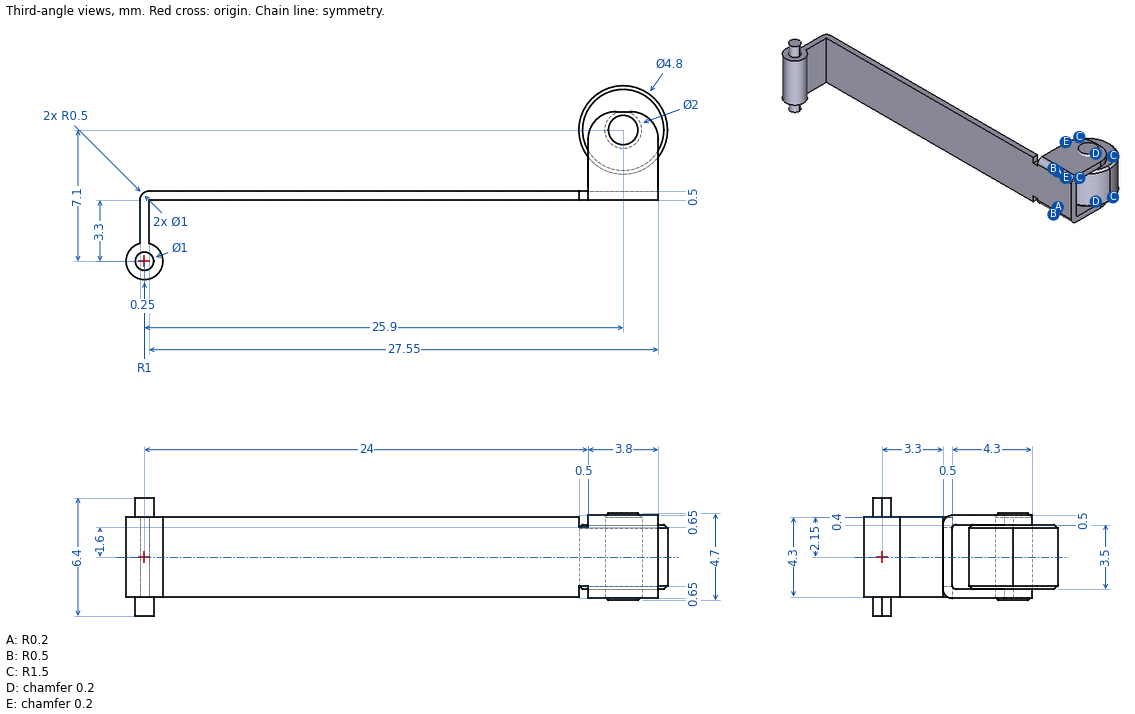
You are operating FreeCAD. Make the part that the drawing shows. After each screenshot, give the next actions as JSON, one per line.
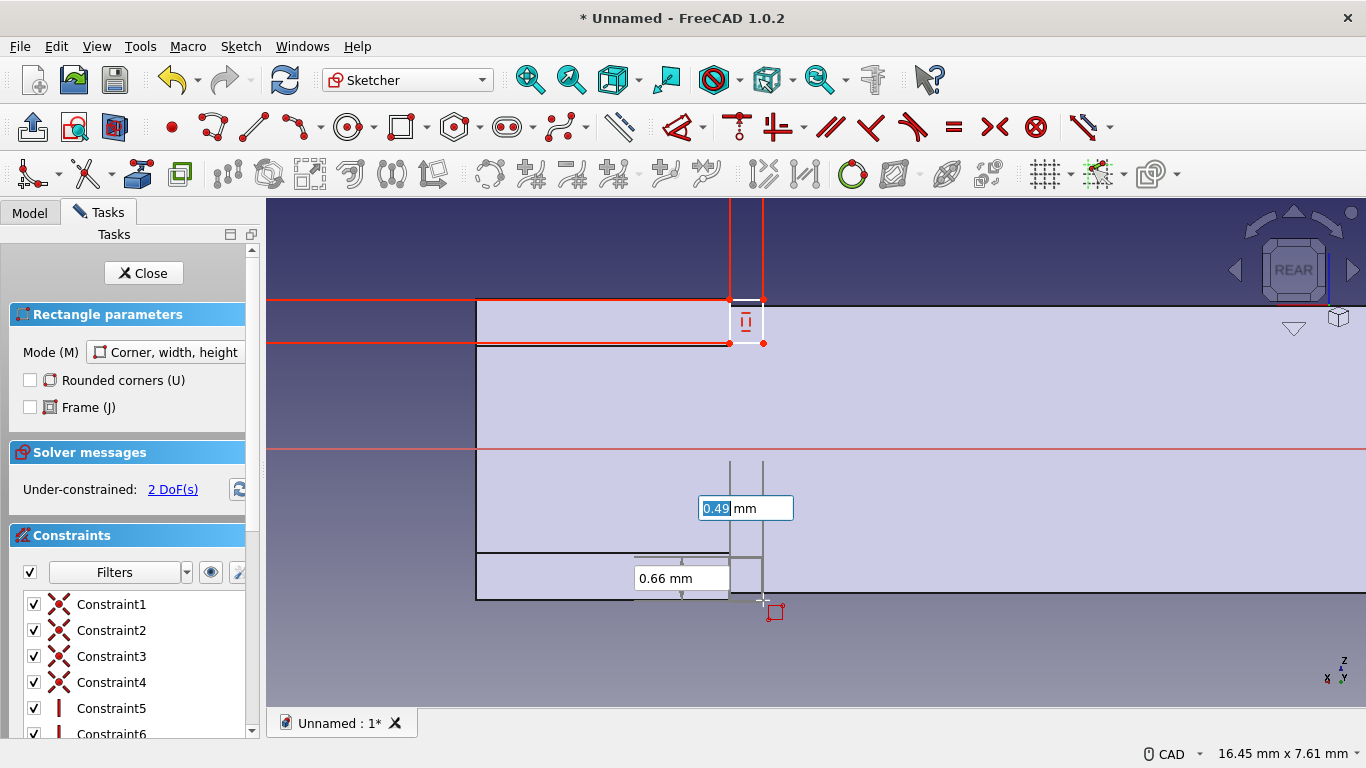
{"action": "type", "text": "0.5"}
{"action": "key", "text": "Tab"}
{"action": "type", "text": "0.65"}
{"action": "key", "text": "Return"}
{"action": "key", "text": "Escape"}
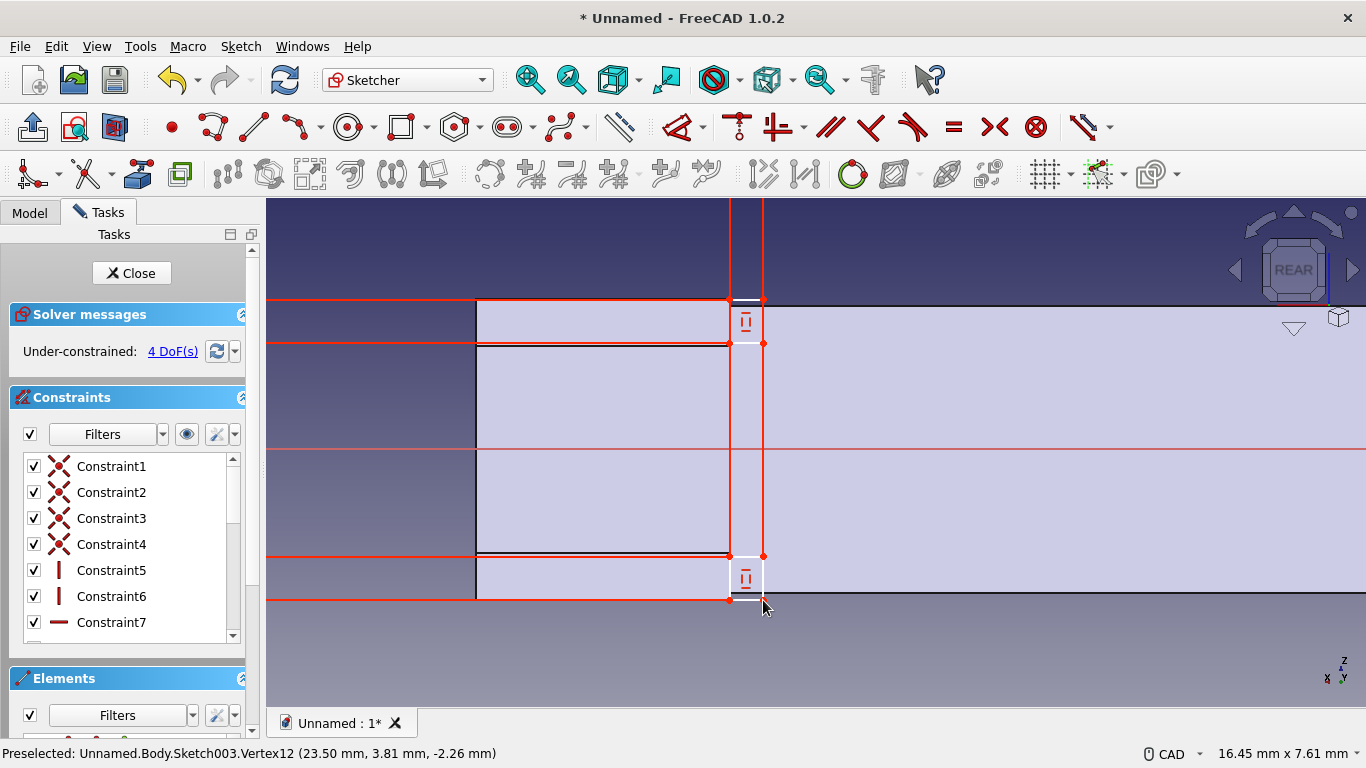
{"action": "left_click", "coordinate": [730, 343]}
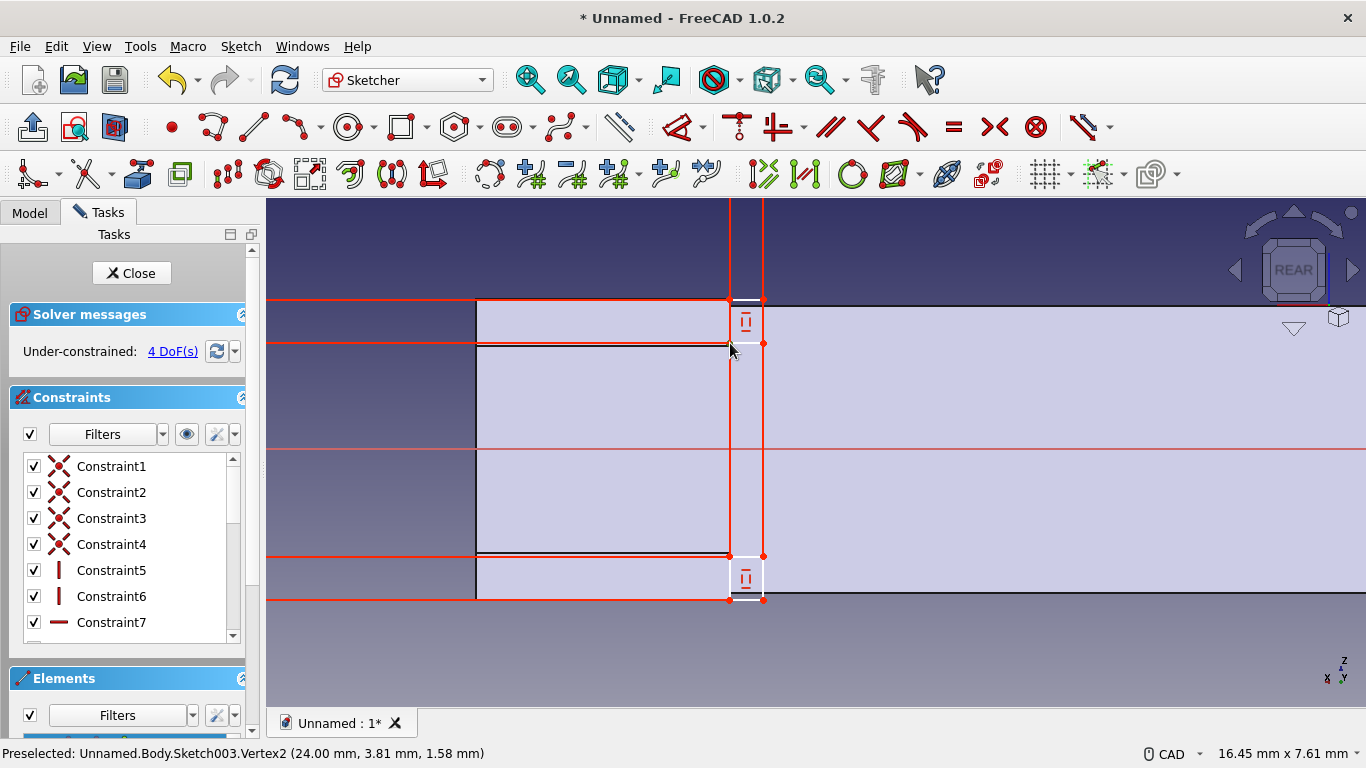
{"action": "left_click", "coordinate": [730, 557]}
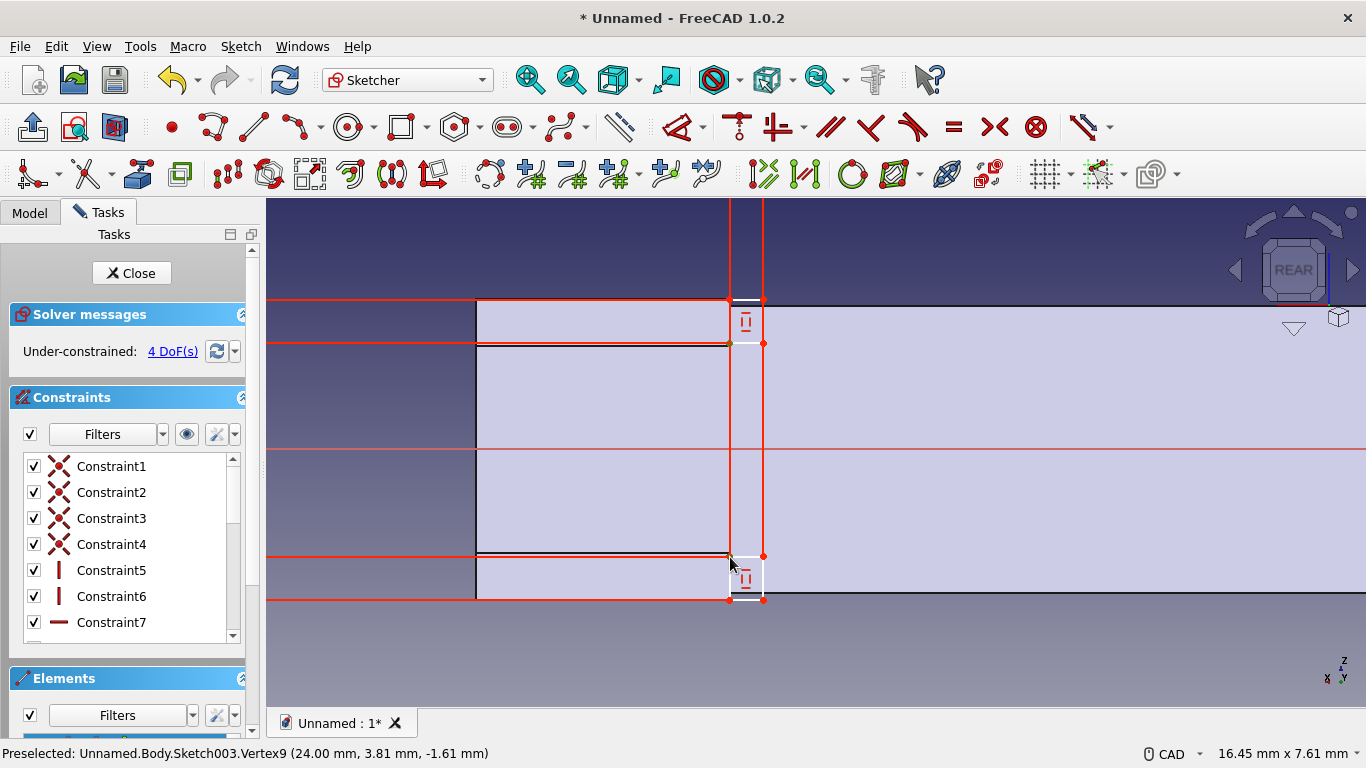
{"action": "left_click", "coordinate": [359, 449]}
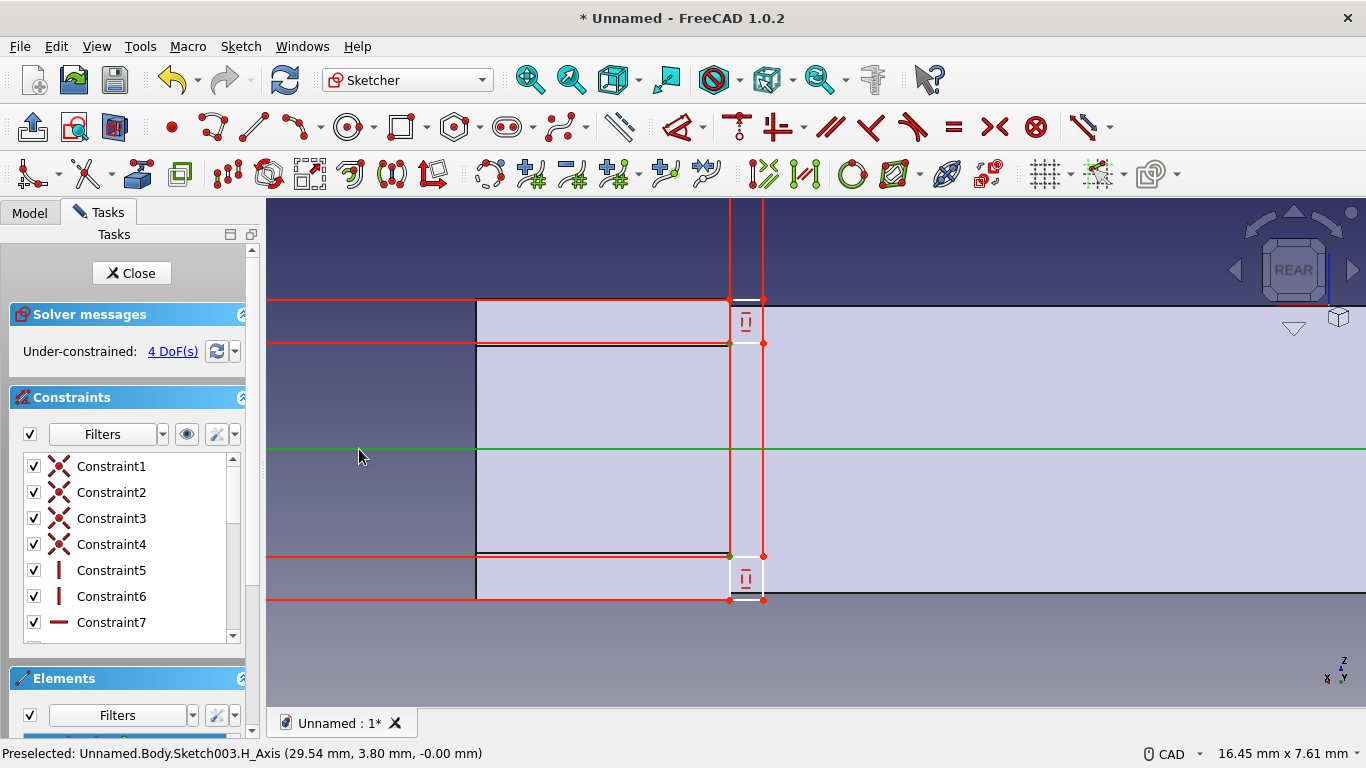
{"action": "key", "text": "s"}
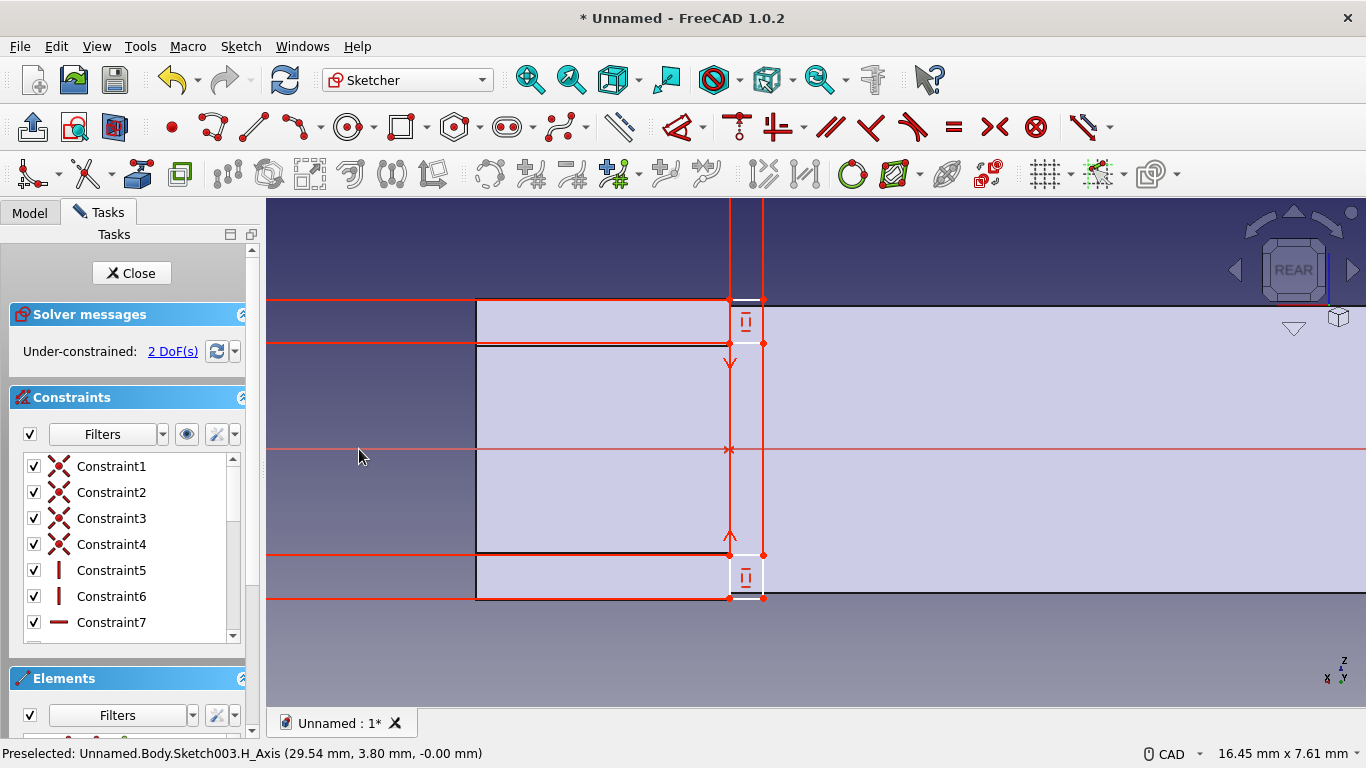
{"action": "key", "text": "d"}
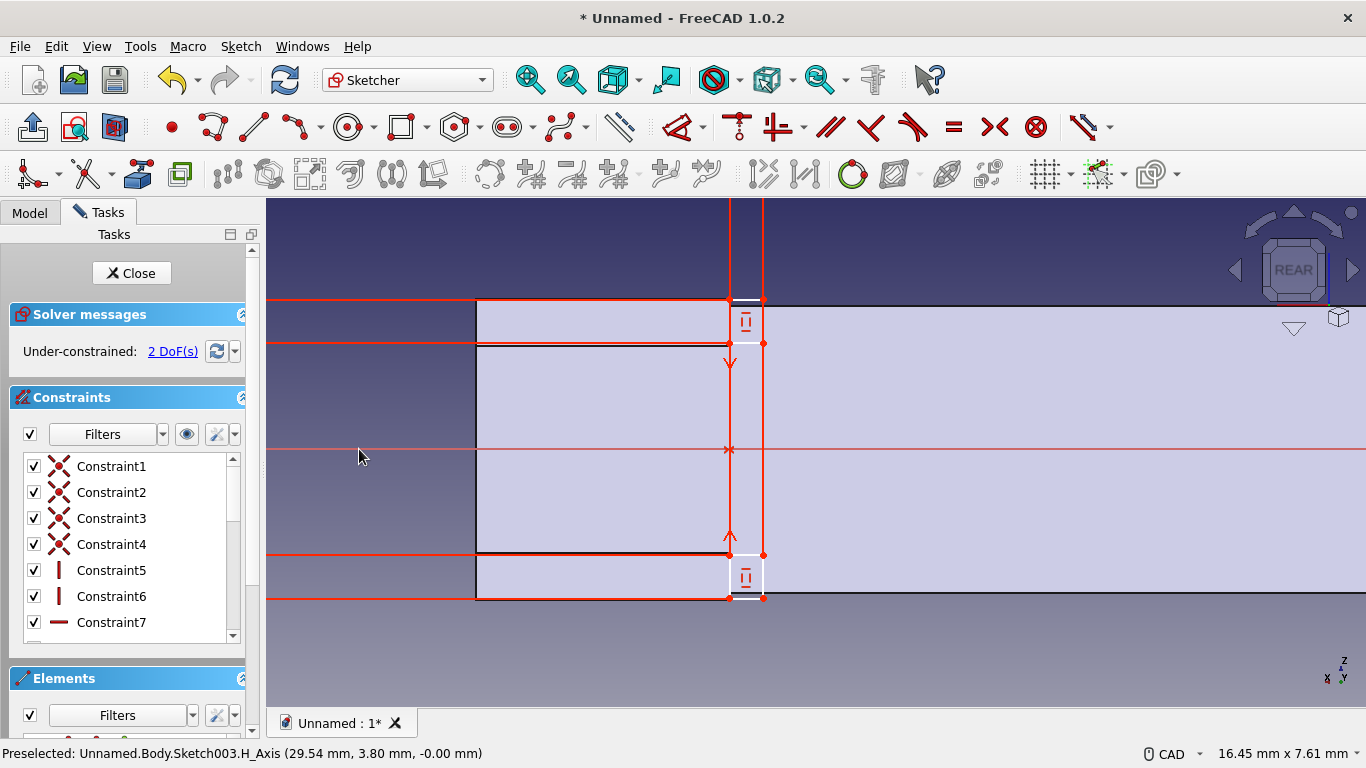
{"action": "left_click", "coordinate": [730, 300]}
{"action": "left_click", "coordinate": [966, 266]}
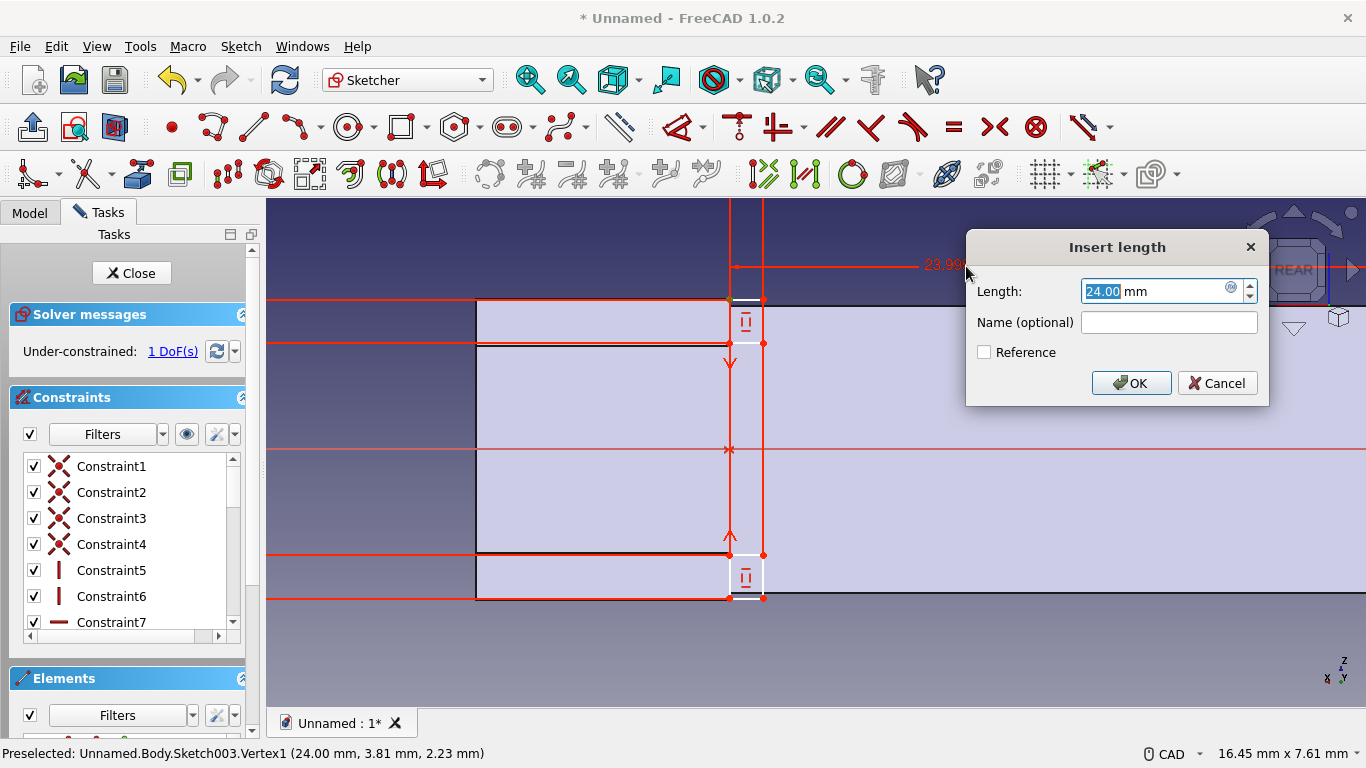
{"action": "type", "text": "24"}
{"action": "key", "text": "Return"}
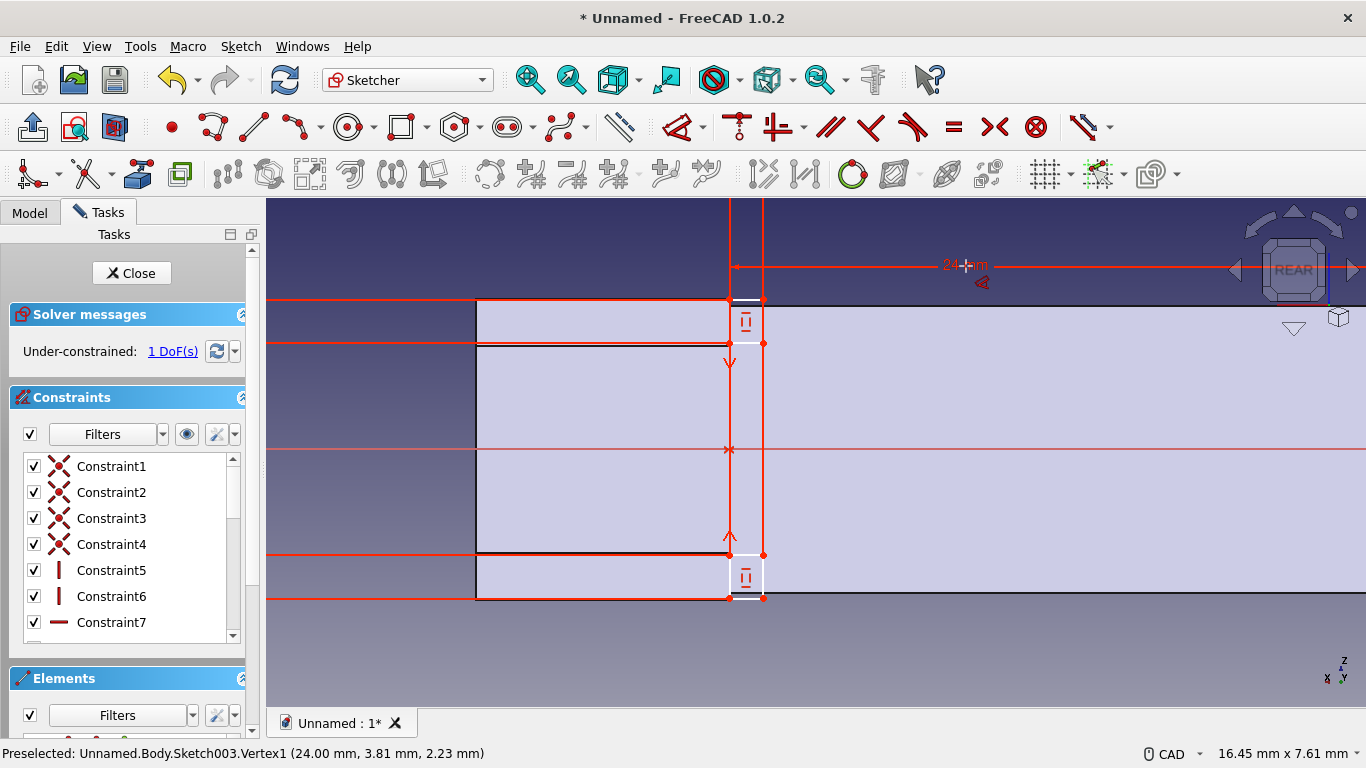
{"action": "left_click", "coordinate": [730, 343]}
{"action": "left_click", "coordinate": [696, 396]}